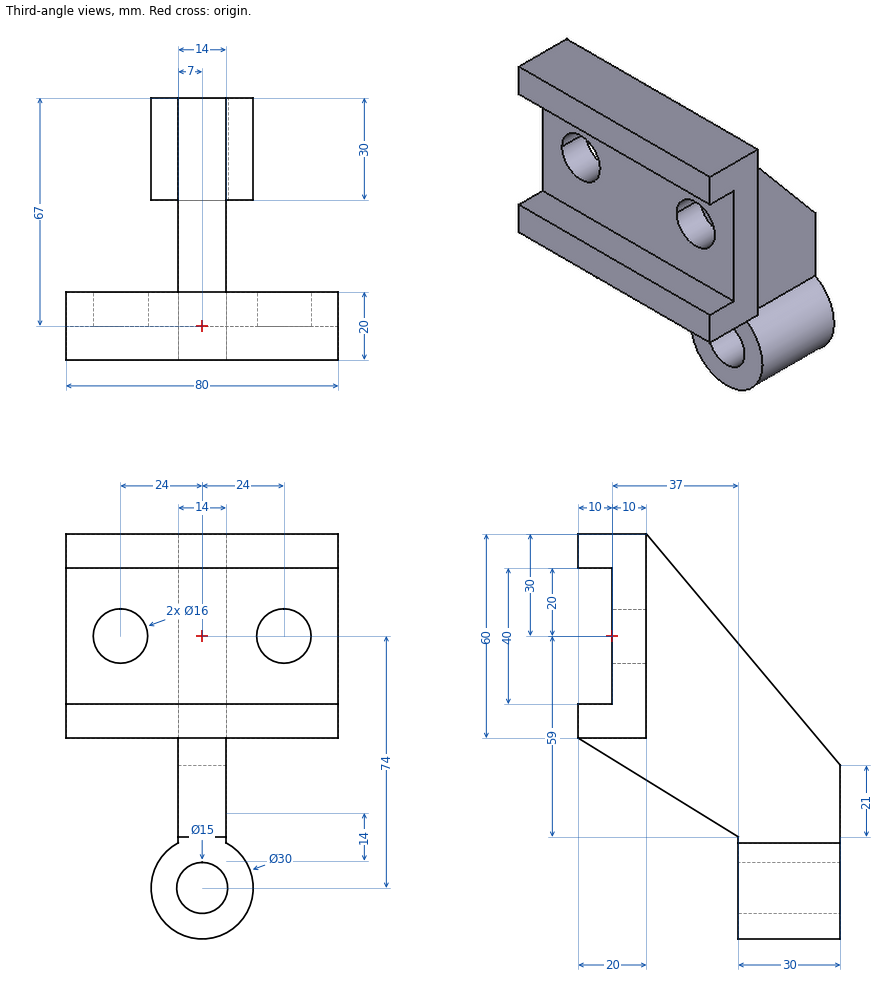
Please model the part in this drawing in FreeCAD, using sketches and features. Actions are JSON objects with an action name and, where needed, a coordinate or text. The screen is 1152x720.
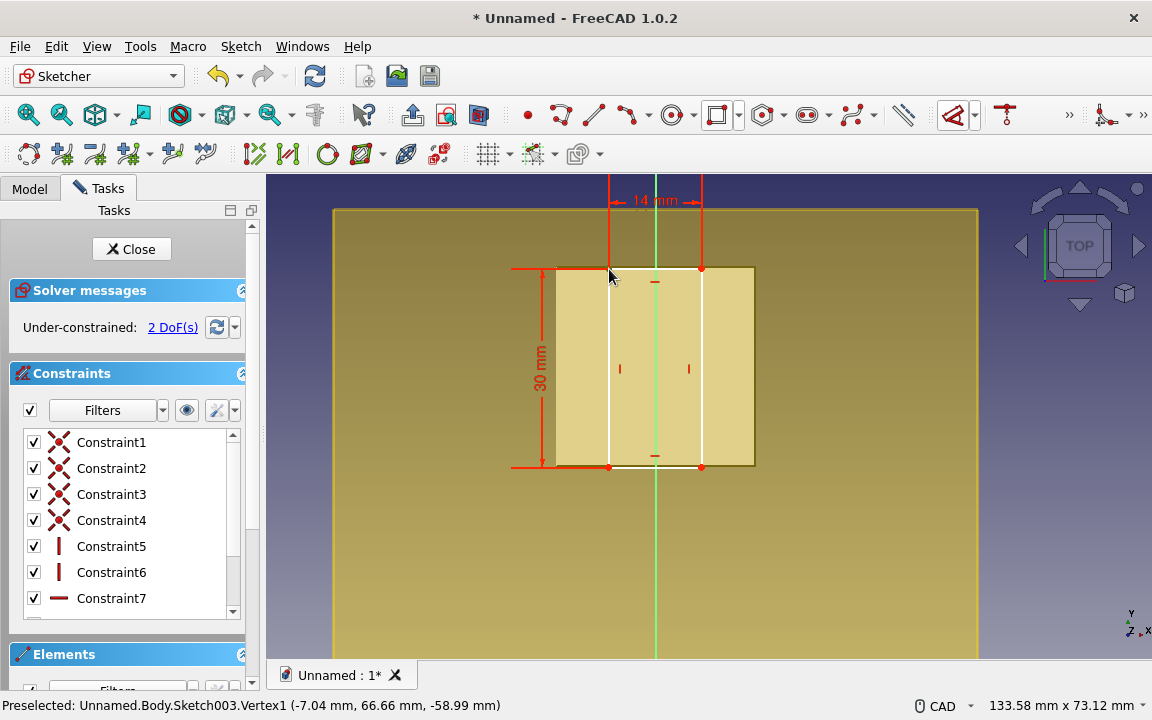
{"action": "left_click", "coordinate": [974, 116]}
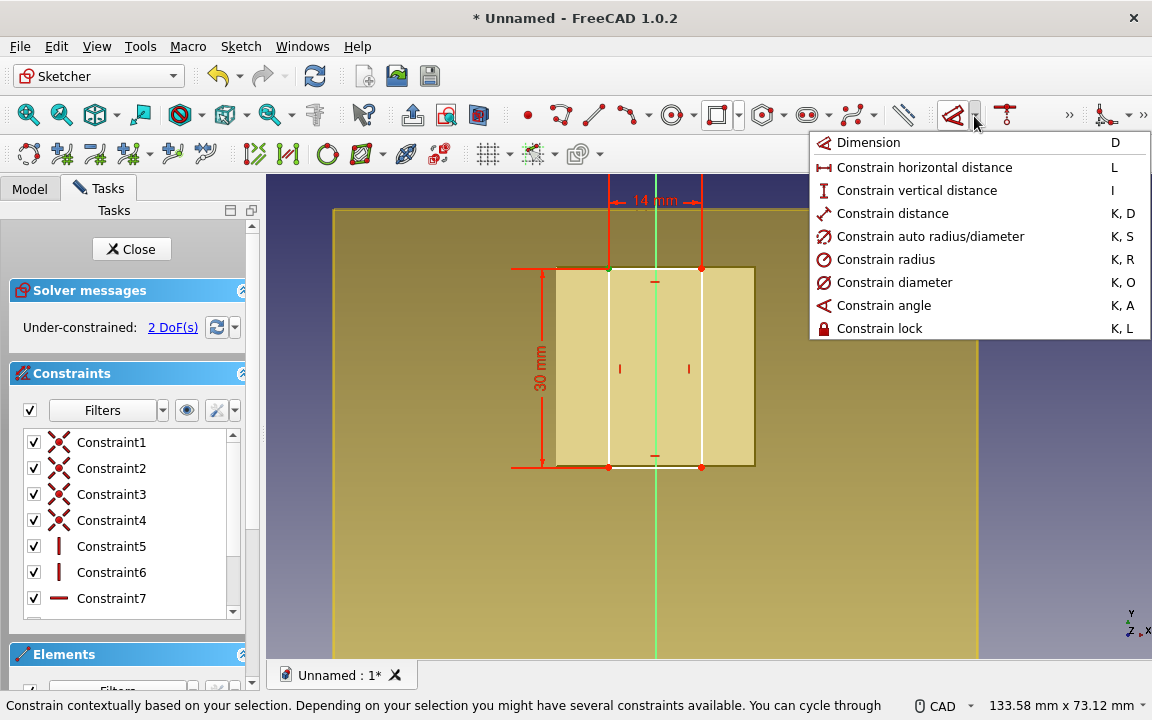
{"action": "left_click", "coordinate": [980, 168]}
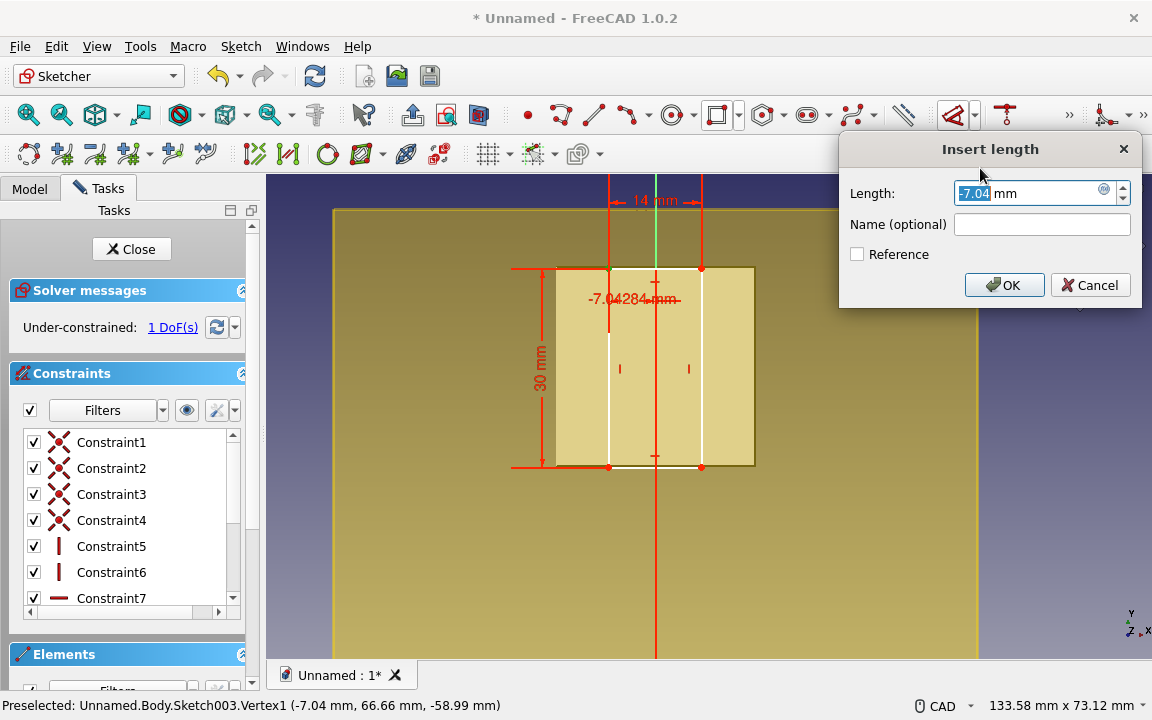
{"action": "type", "text": "-7"}
{"action": "key", "text": "Return"}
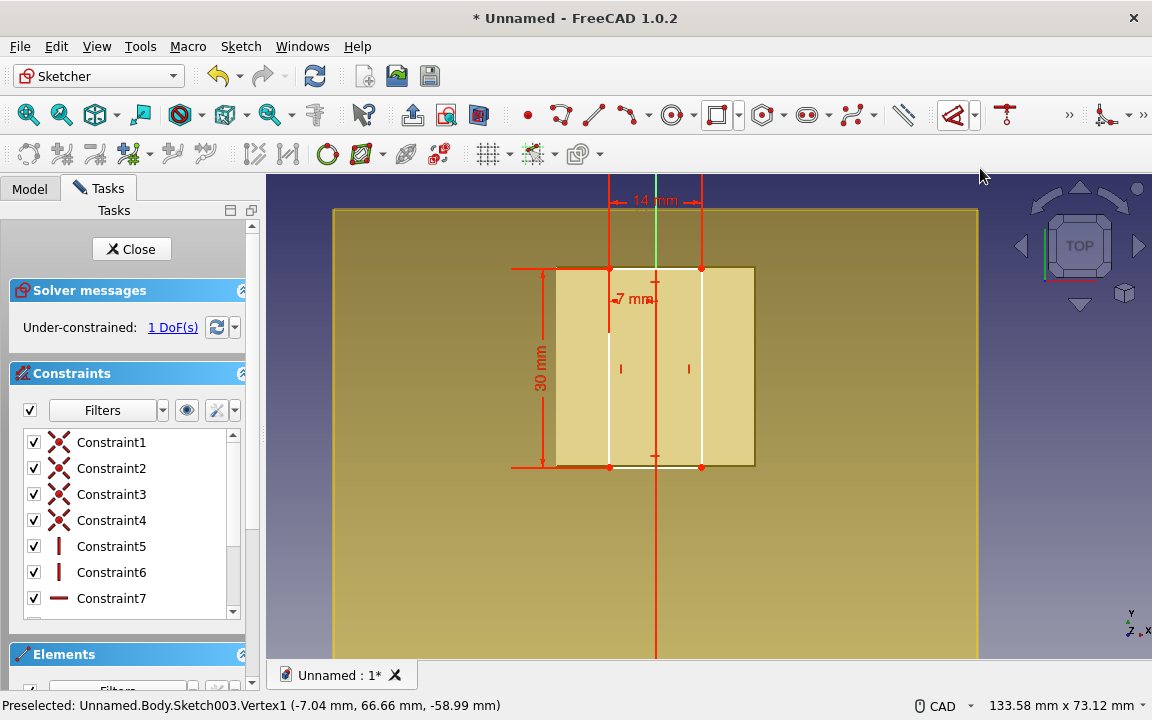
{"action": "left_click", "coordinate": [609, 269]}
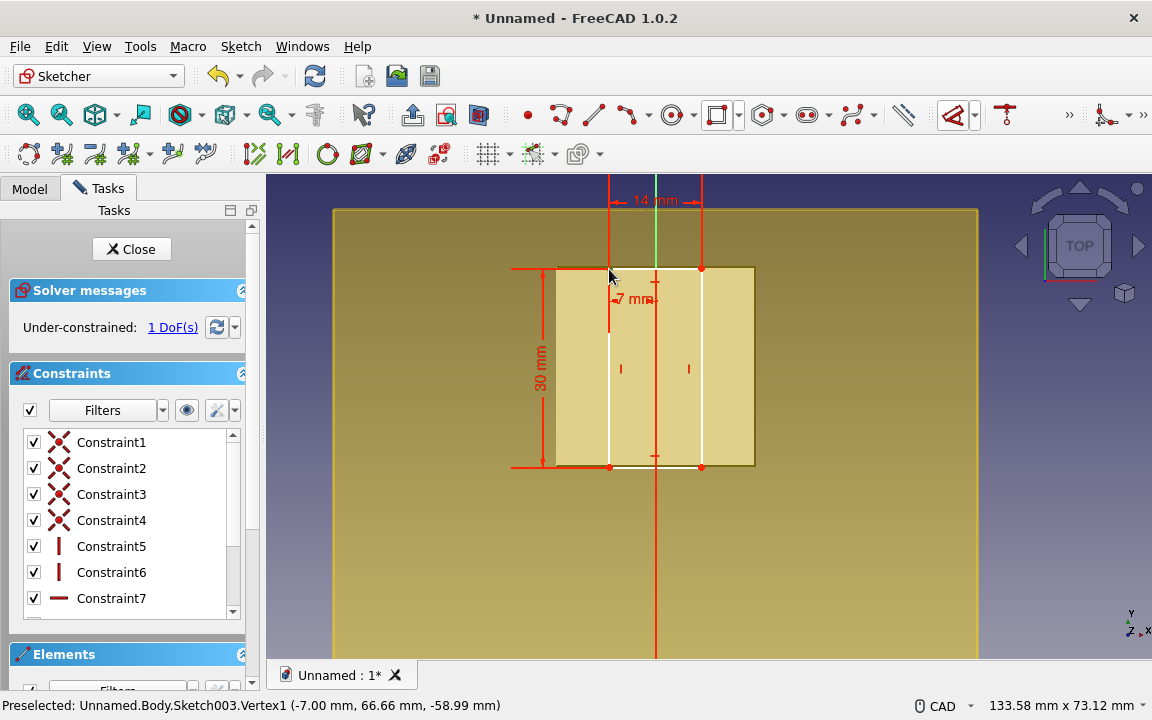
{"action": "left_click", "coordinate": [974, 116]}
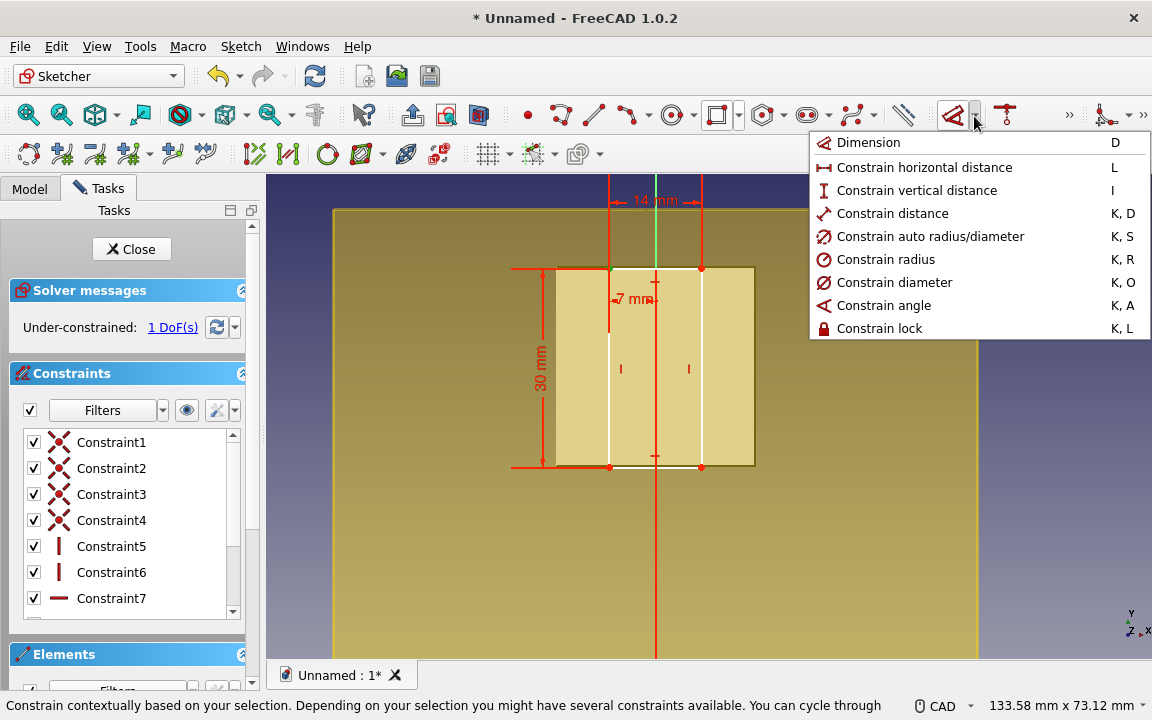
{"action": "left_click", "coordinate": [980, 190]}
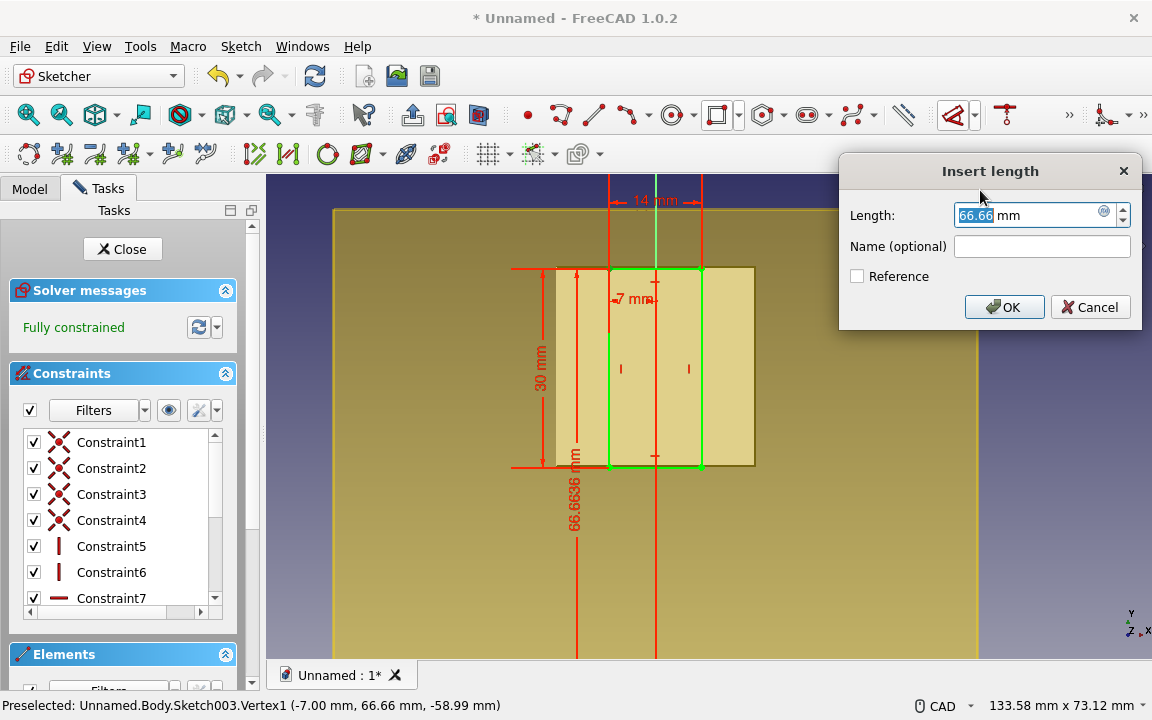
{"action": "type", "text": "67"}
{"action": "key", "text": "Return"}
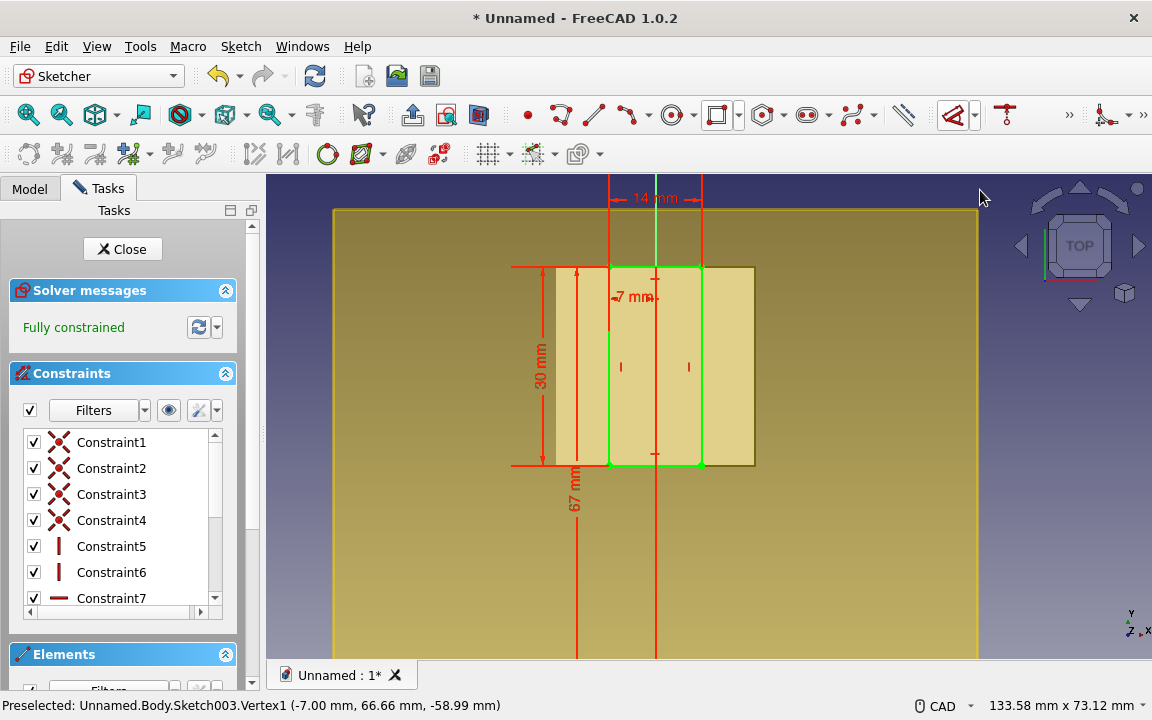
{"action": "left_click", "coordinate": [123, 249]}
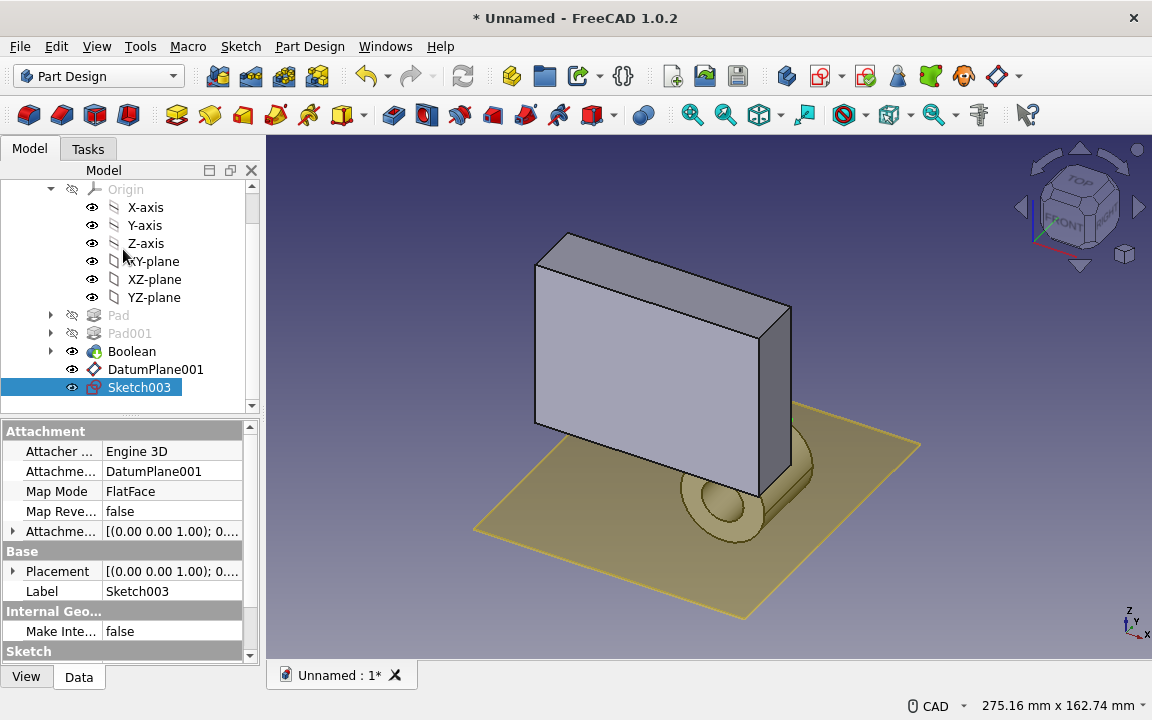
{"action": "left_click", "coordinate": [177, 116]}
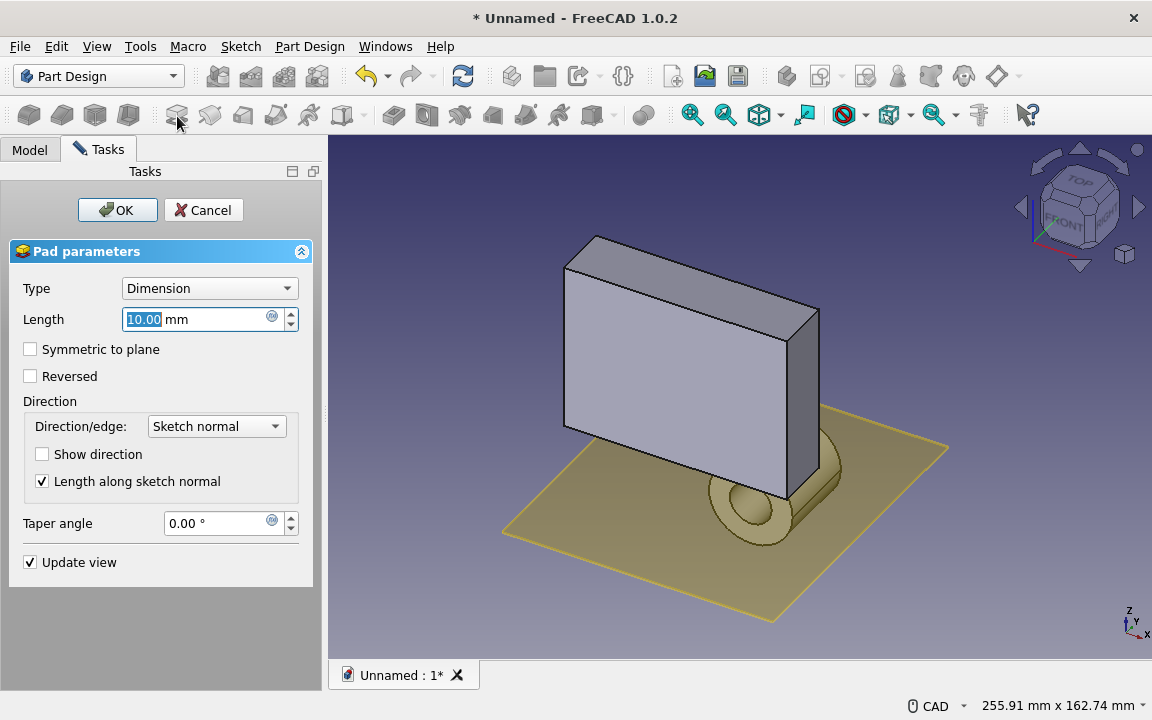
{"action": "type", "text": "14"}
{"action": "key", "text": "Tab"}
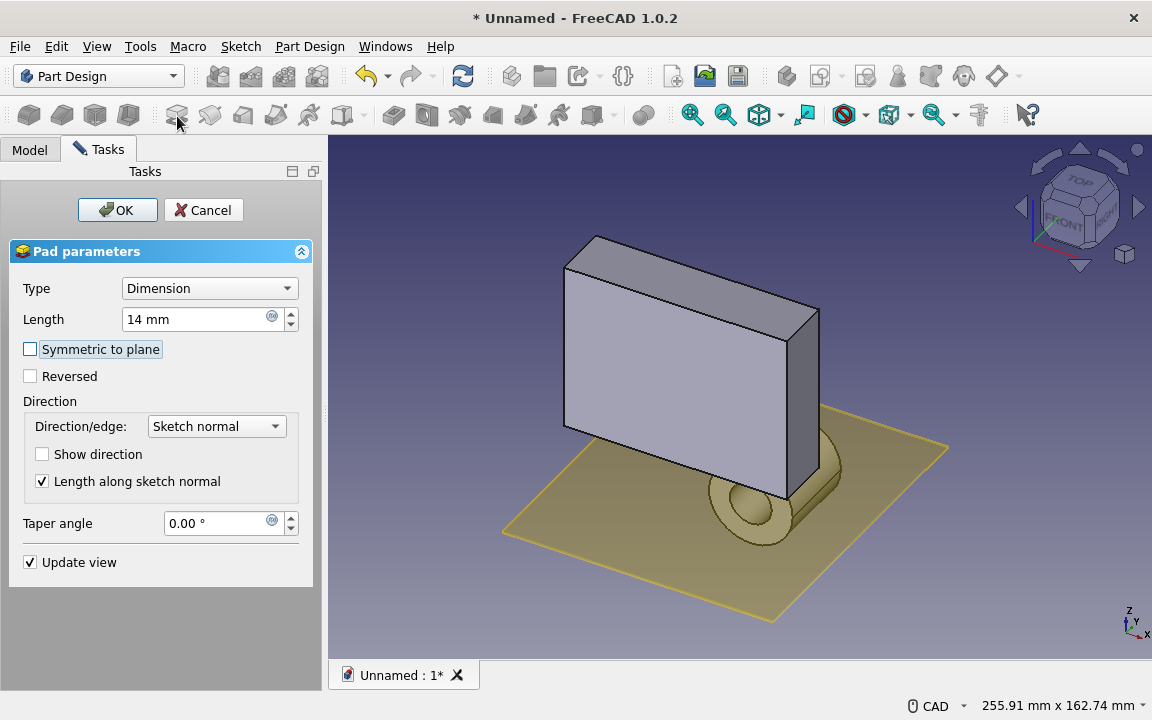
{"action": "left_click", "coordinate": [31, 349]}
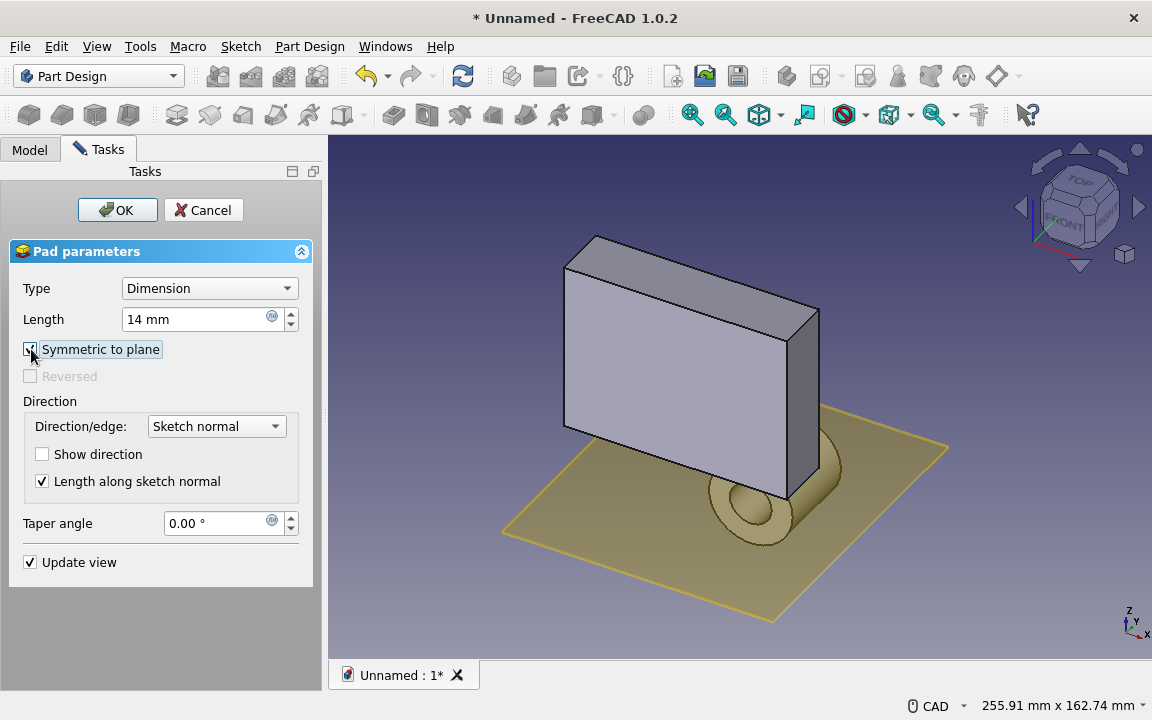
{"action": "left_click", "coordinate": [118, 210]}